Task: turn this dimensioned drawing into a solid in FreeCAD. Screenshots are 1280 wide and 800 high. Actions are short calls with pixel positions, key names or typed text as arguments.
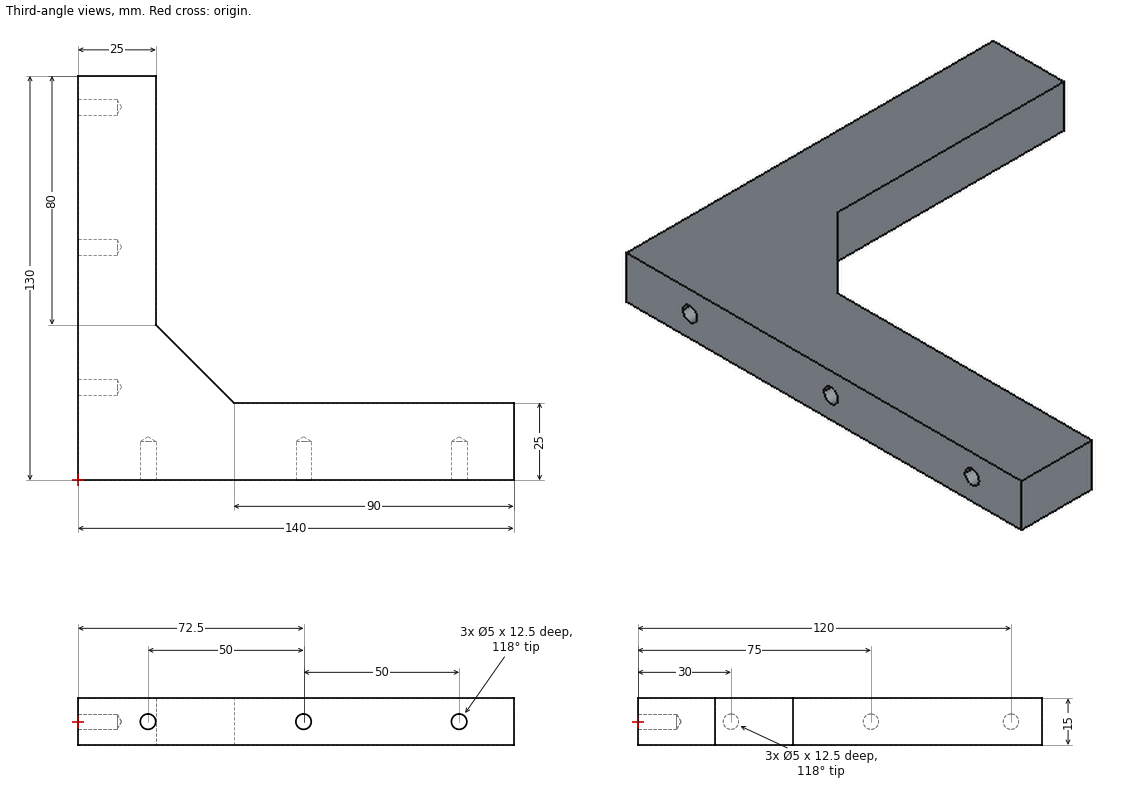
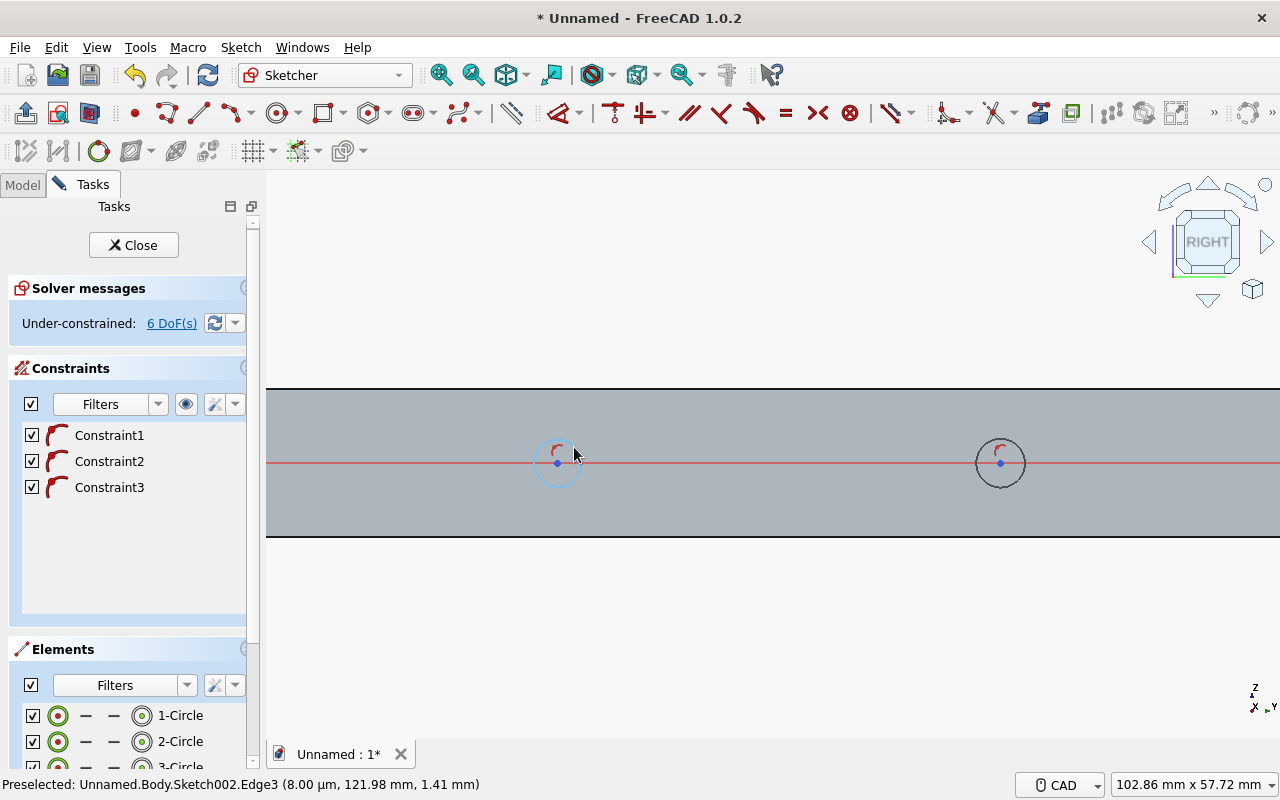
click(574, 446)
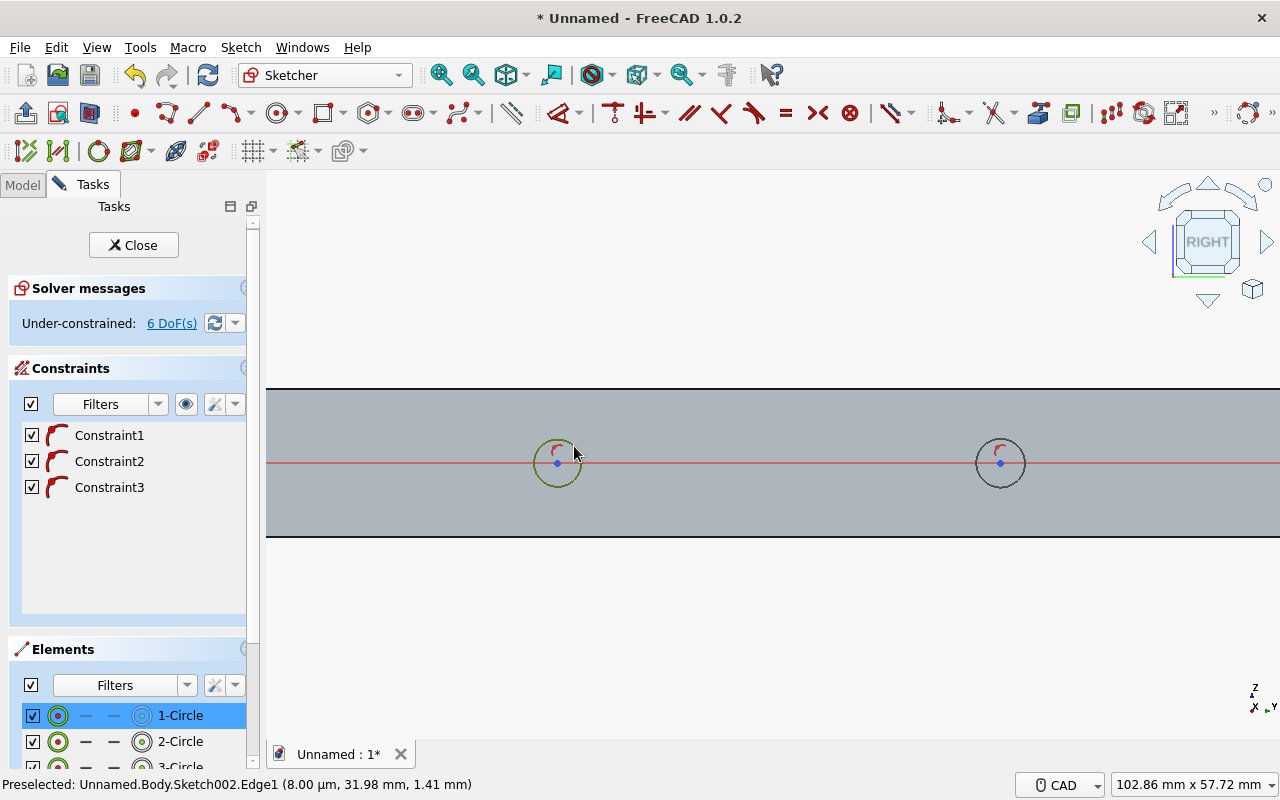
click(1018, 446)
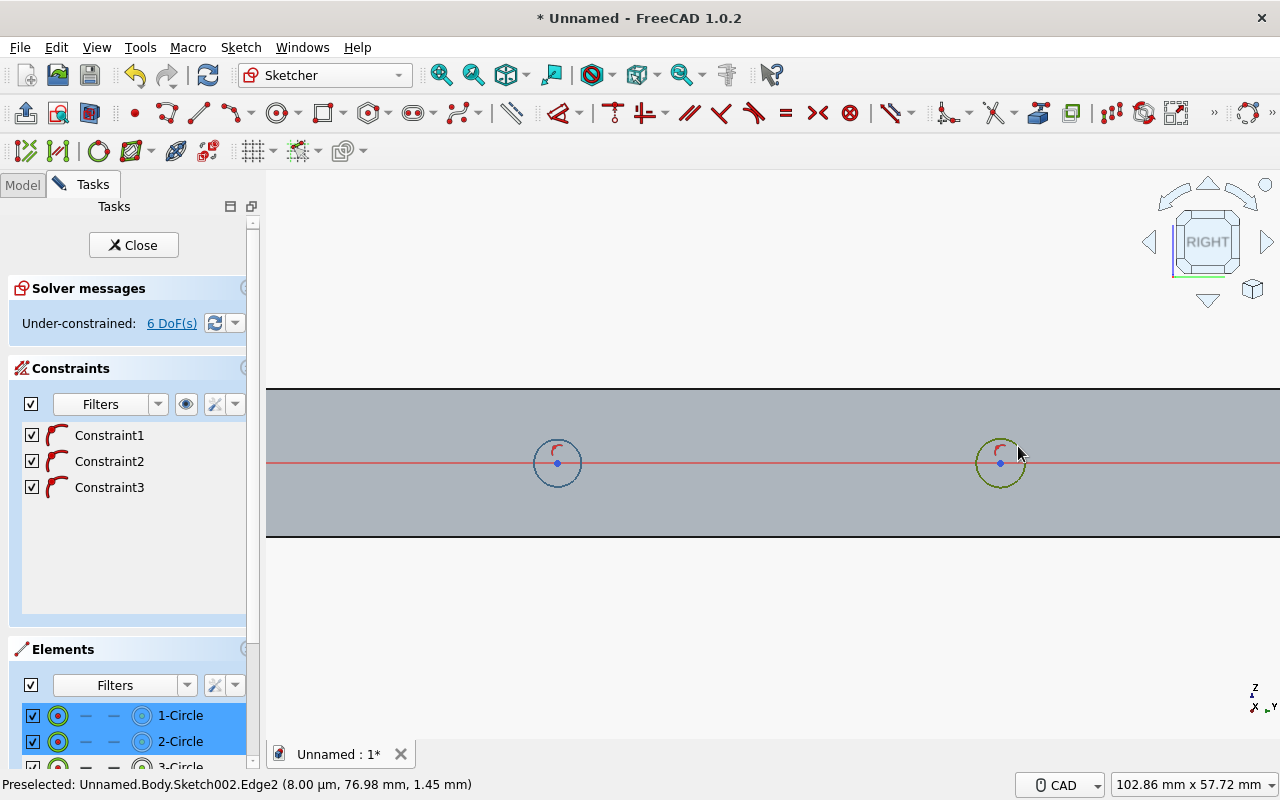
scroll(573, 447, down, 4)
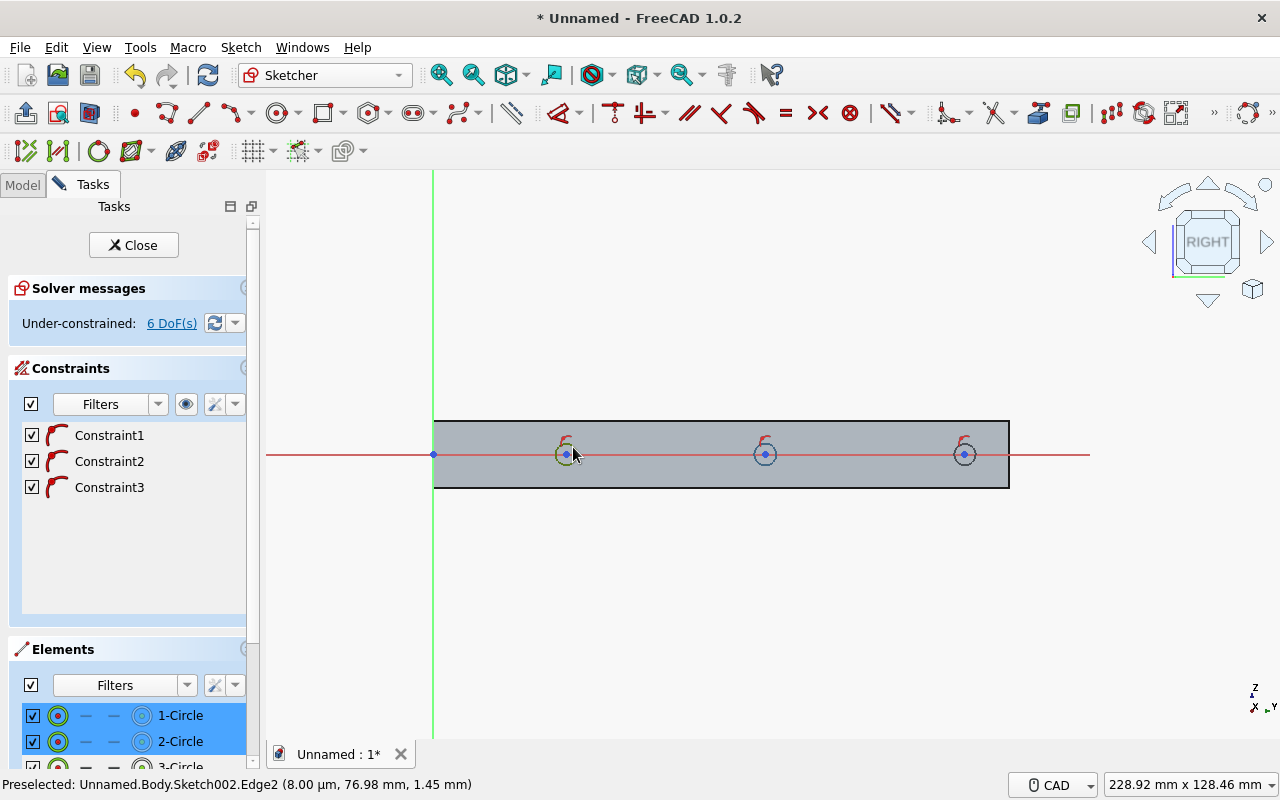
scroll(972, 447, up, 4)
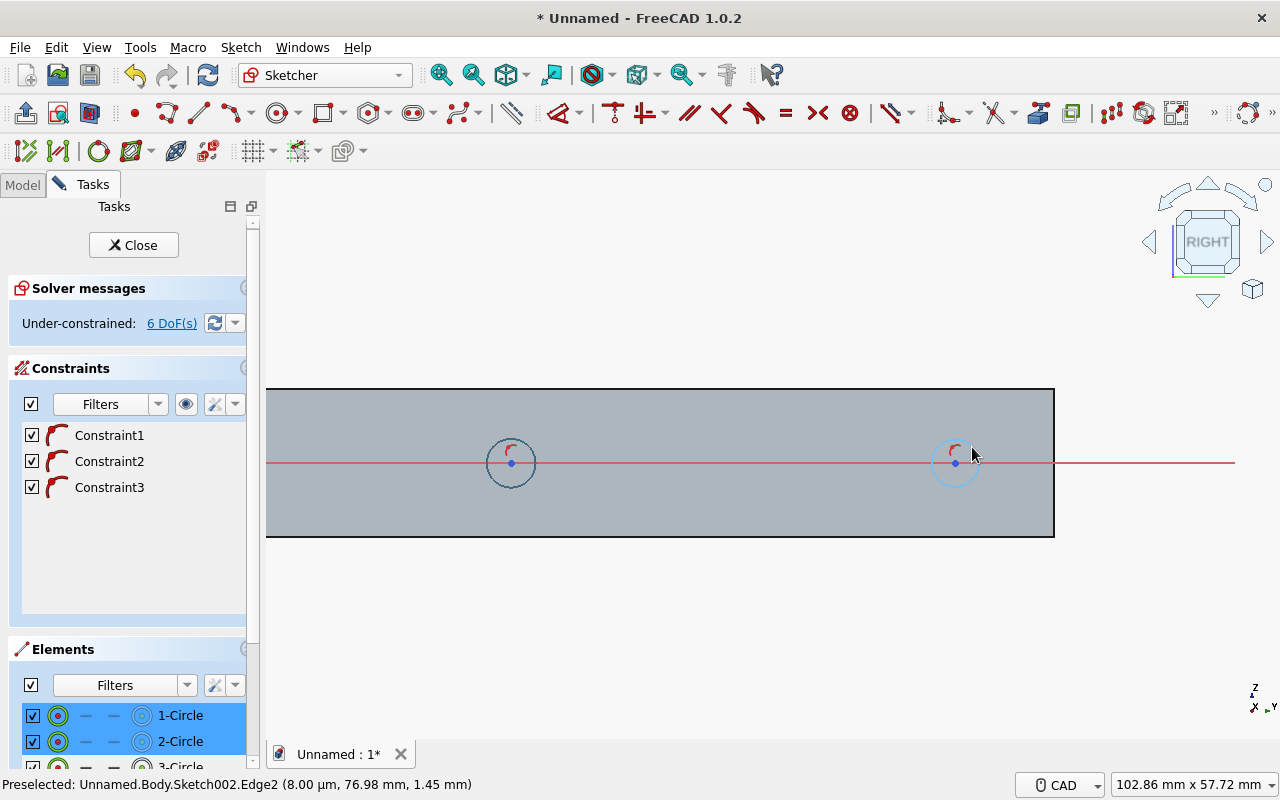
click(972, 446)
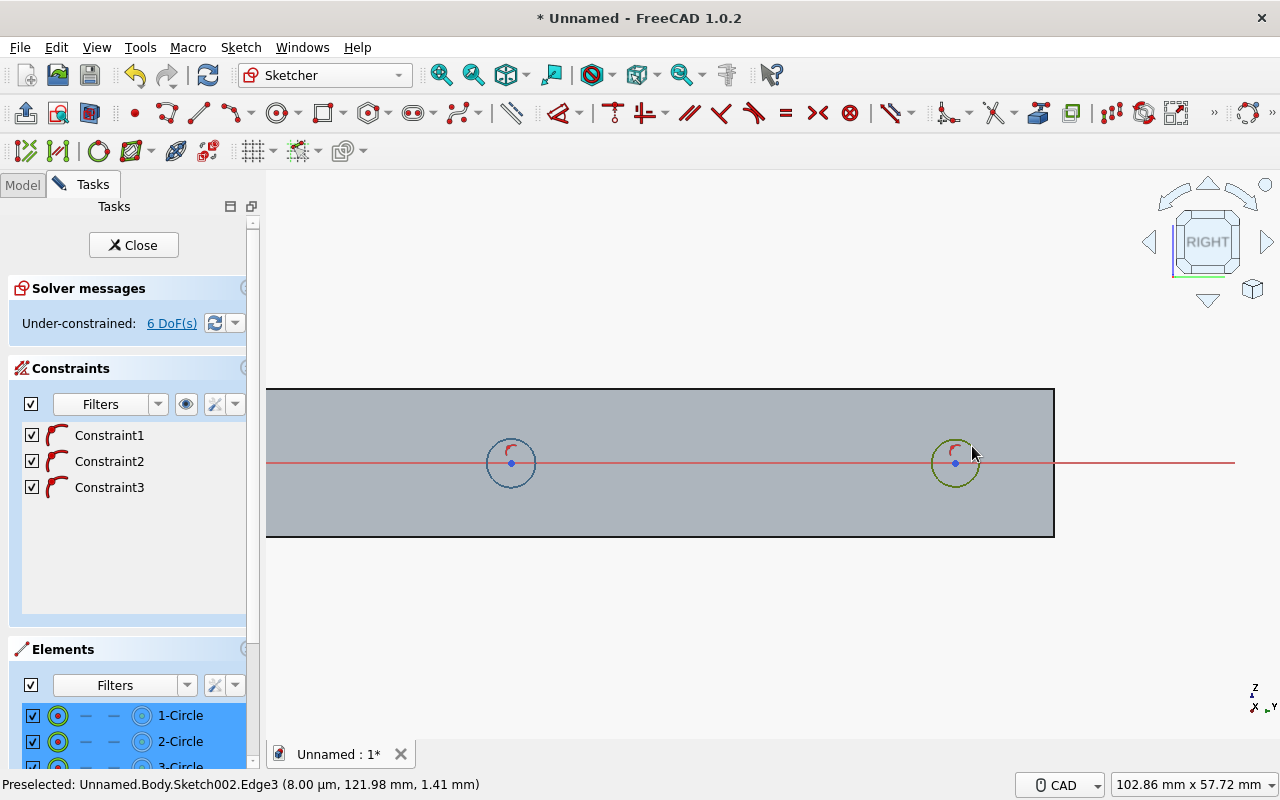
click(786, 114)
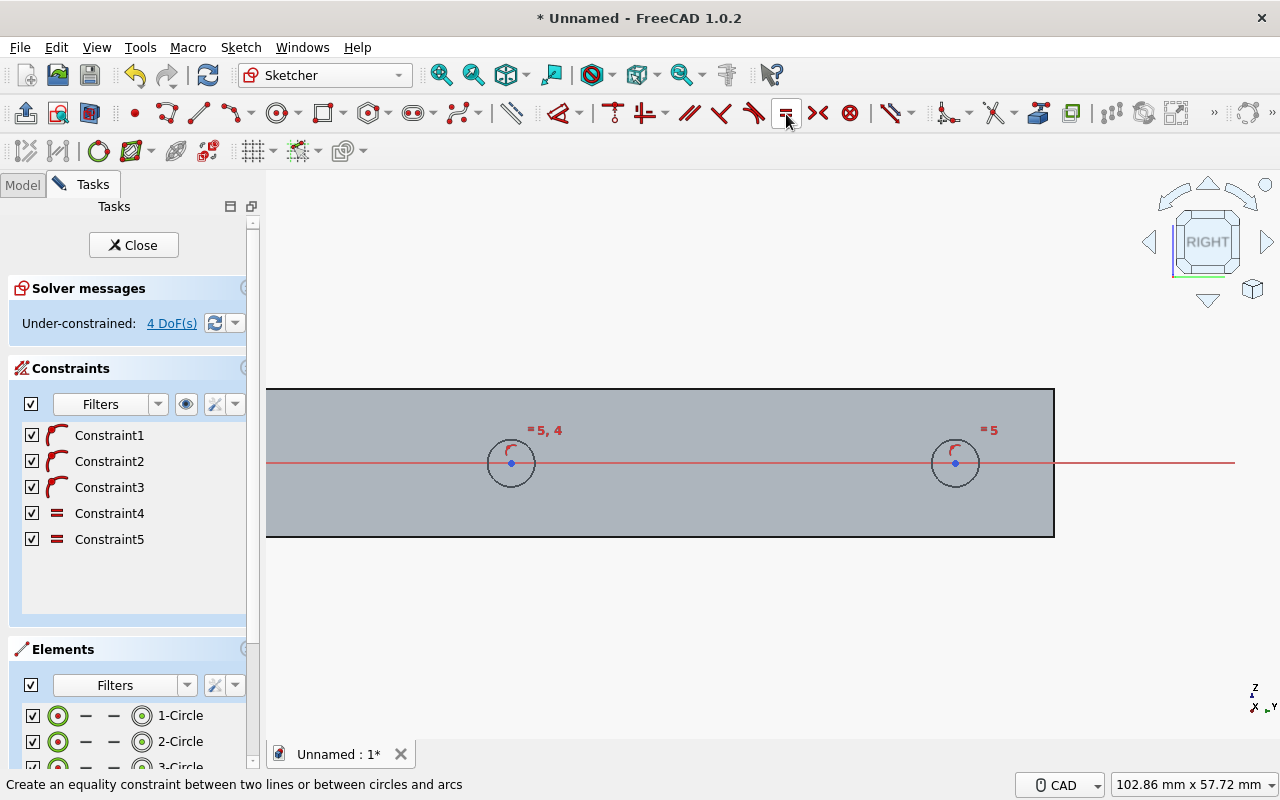
click(558, 114)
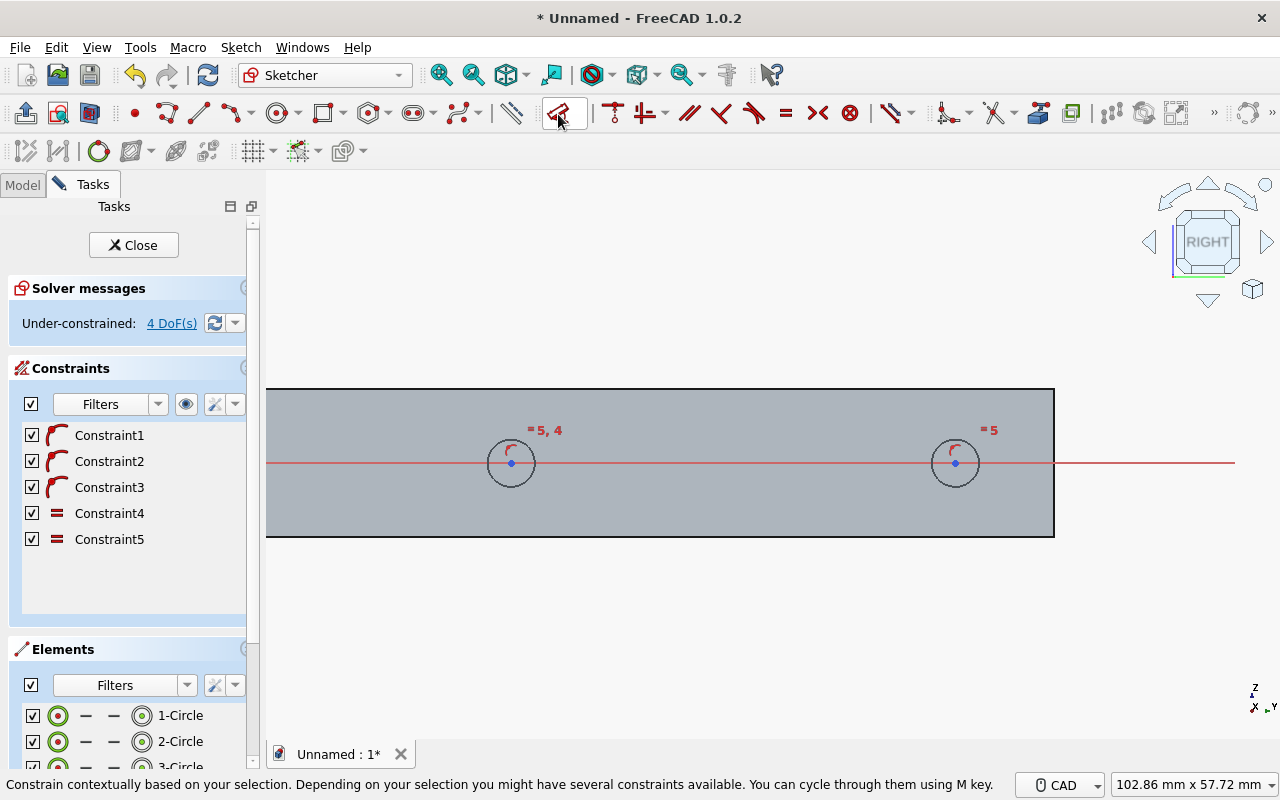
scroll(973, 447, down, 4)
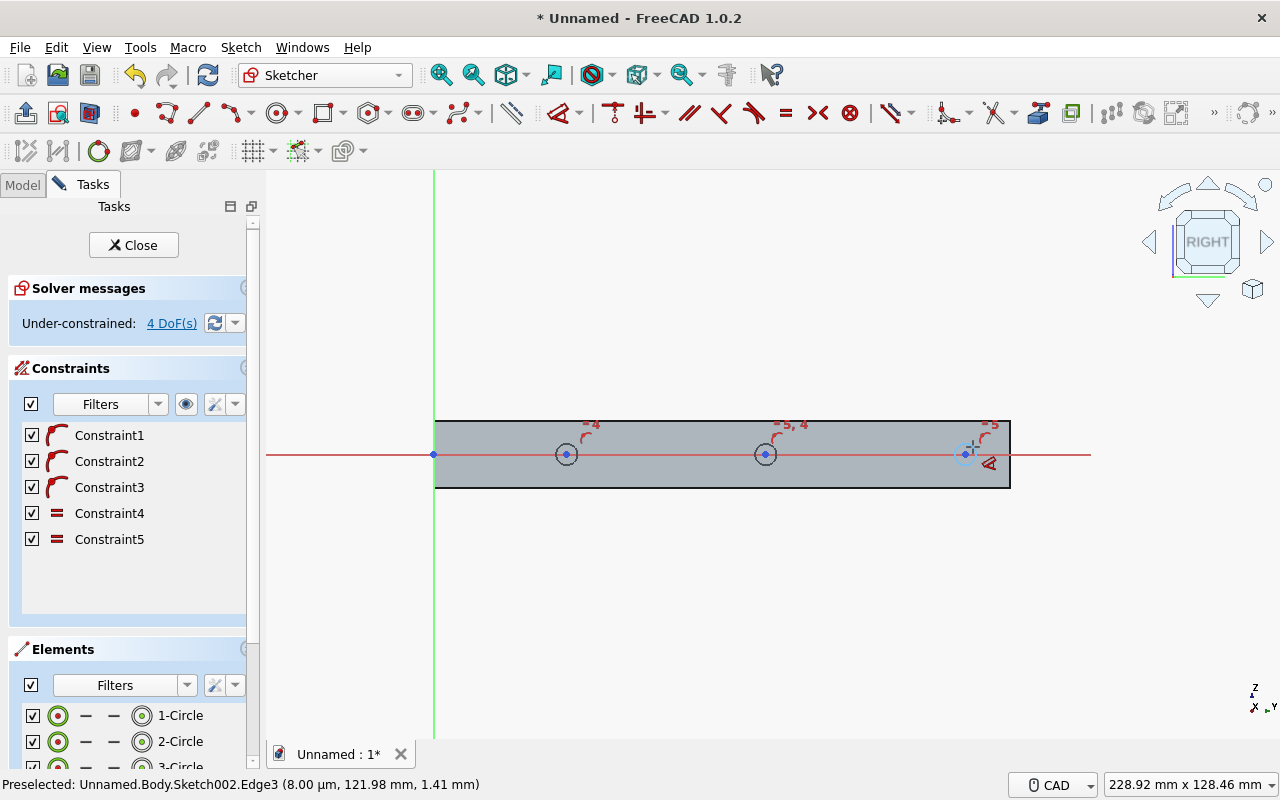
scroll(574, 447, up, 4)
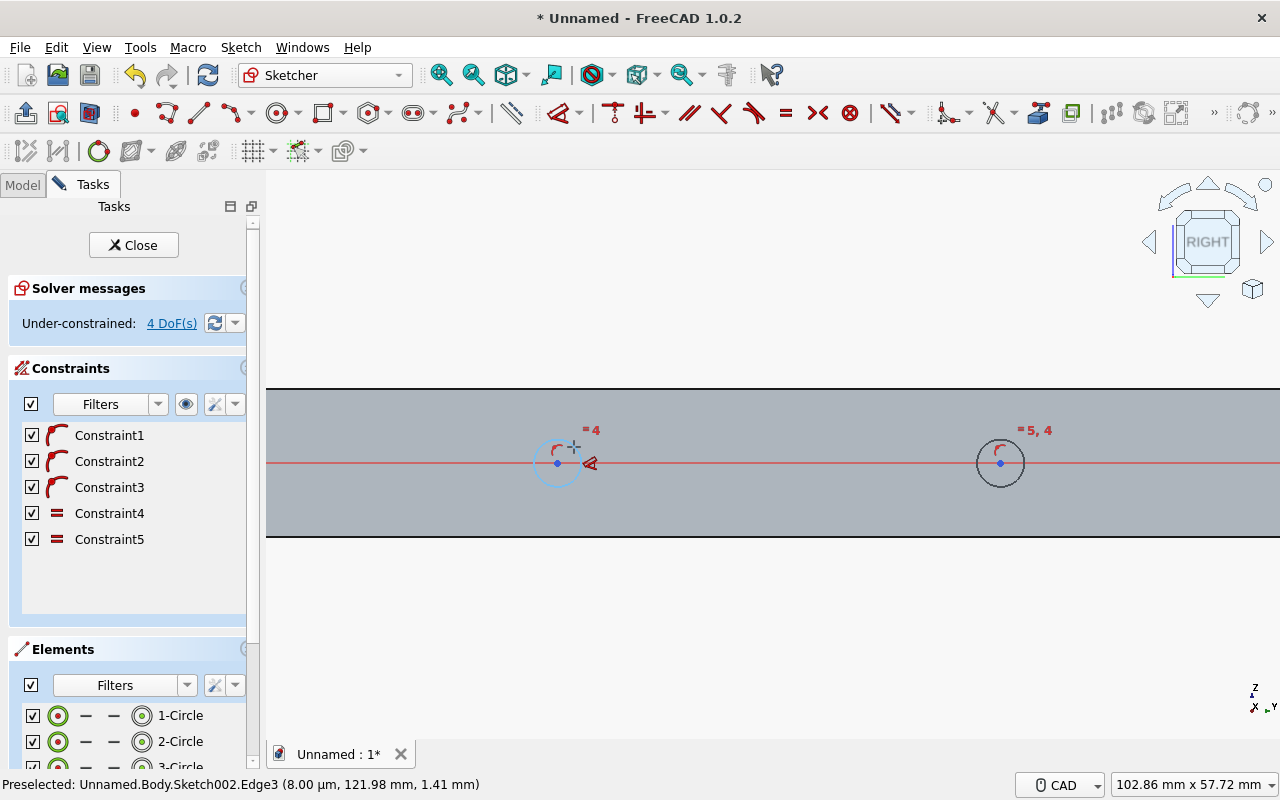
click(574, 446)
click(596, 423)